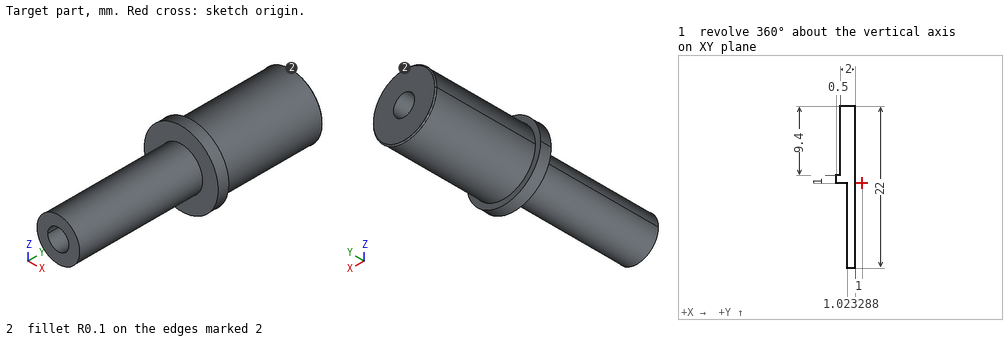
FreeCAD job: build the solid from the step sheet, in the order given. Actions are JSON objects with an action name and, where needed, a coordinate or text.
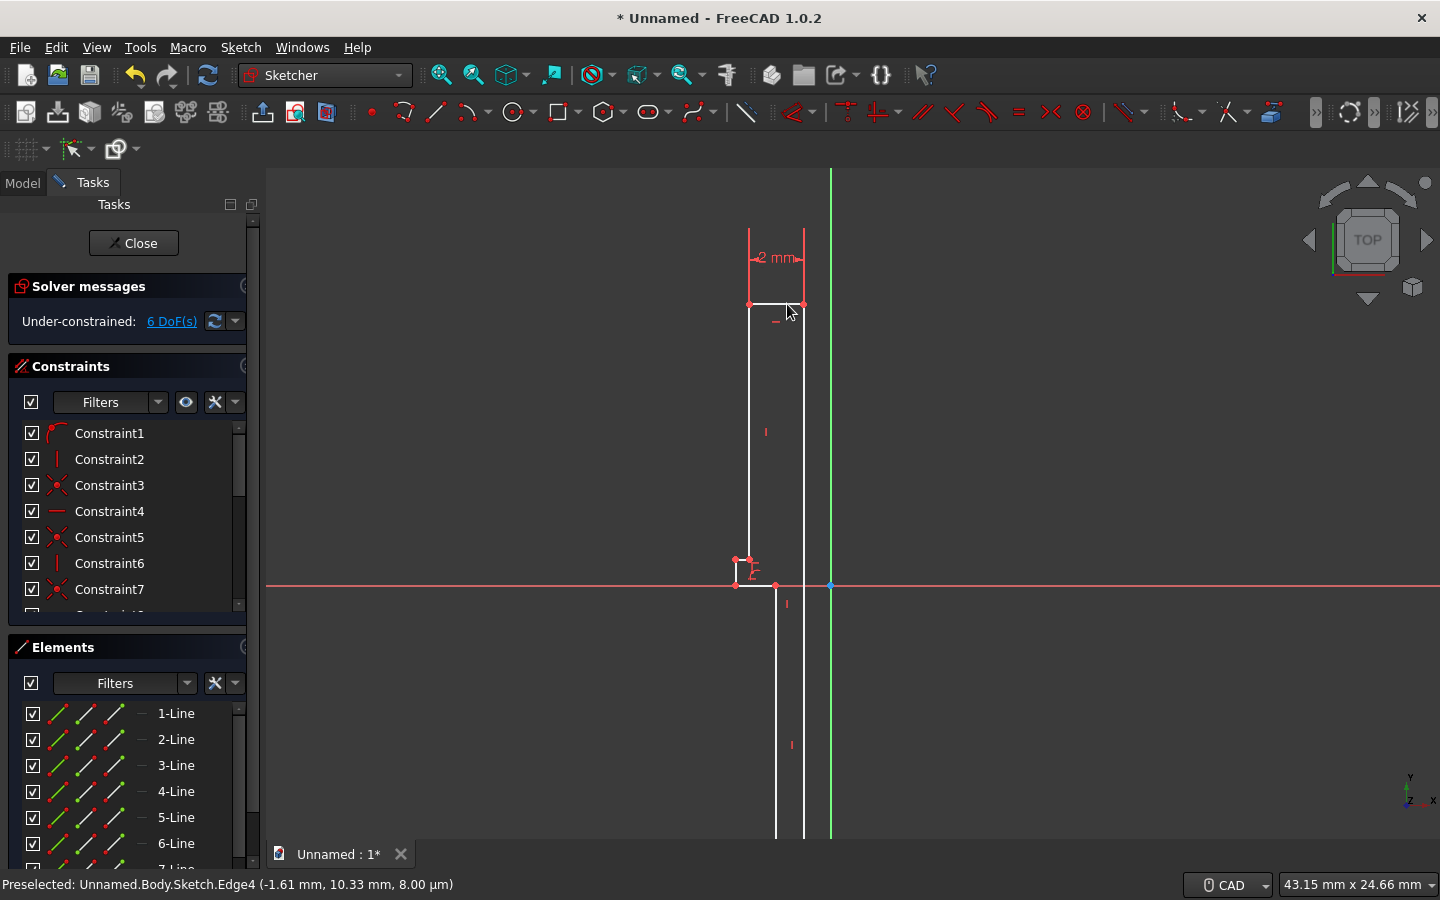
{"action": "scroll", "coordinate": [736, 570], "scroll_direction": "up", "scroll_amount": 2}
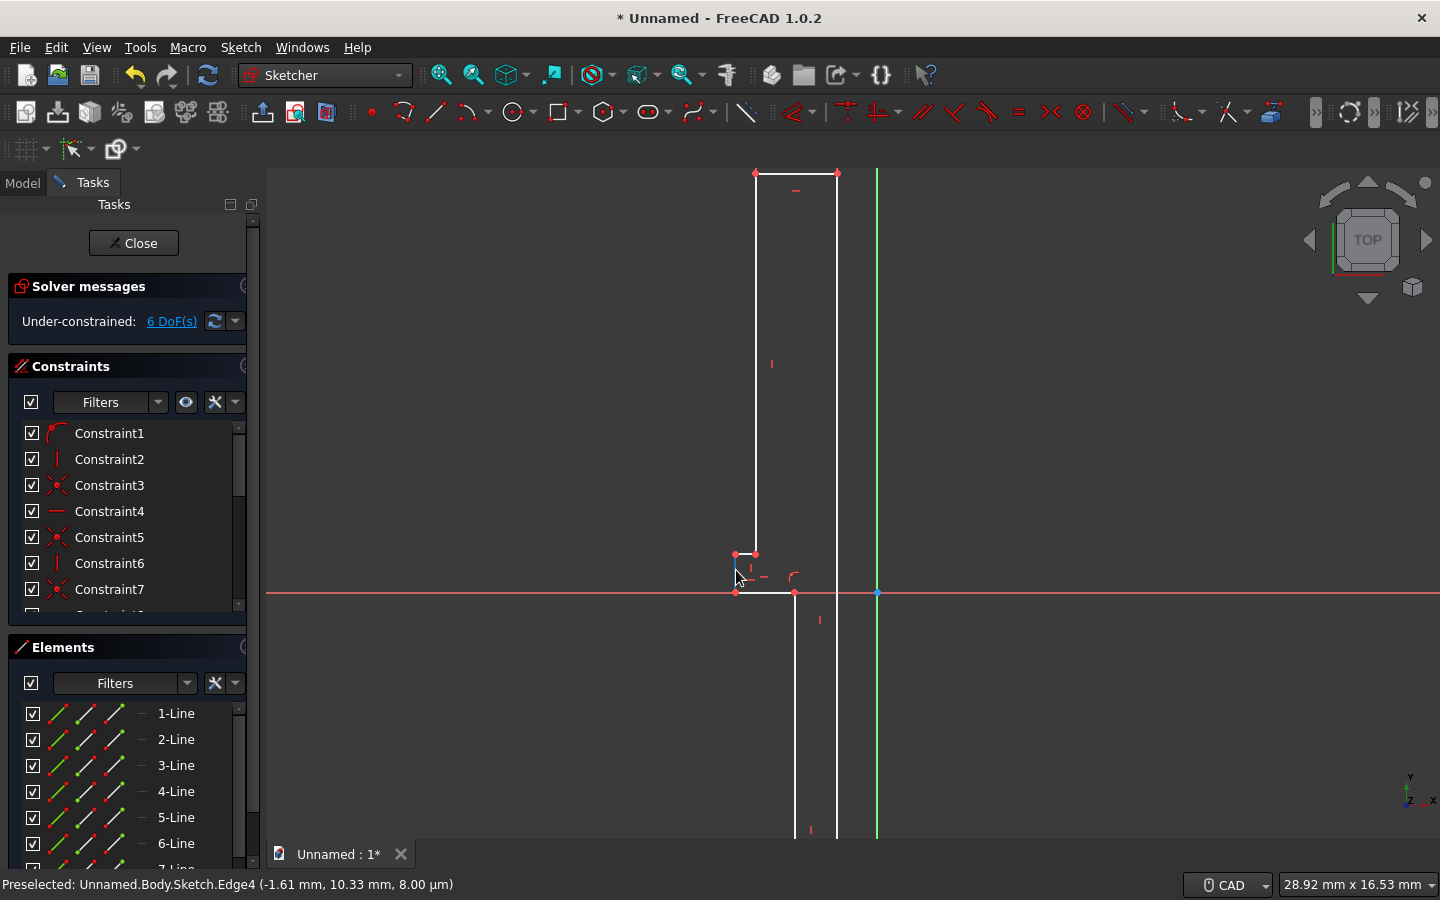
{"action": "left_click", "coordinate": [735, 570]}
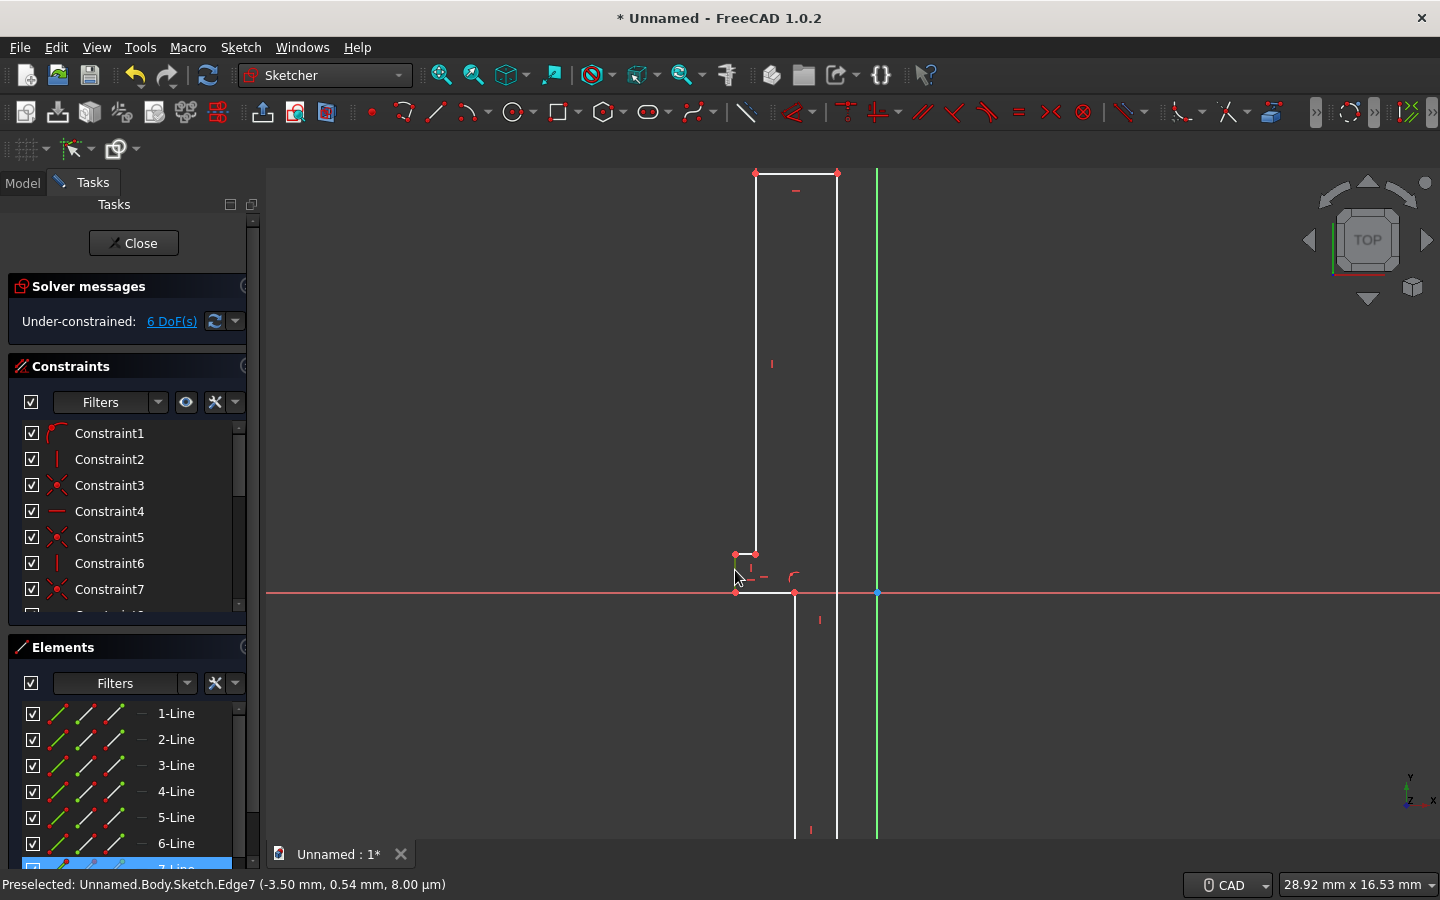
{"action": "key", "text": "i"}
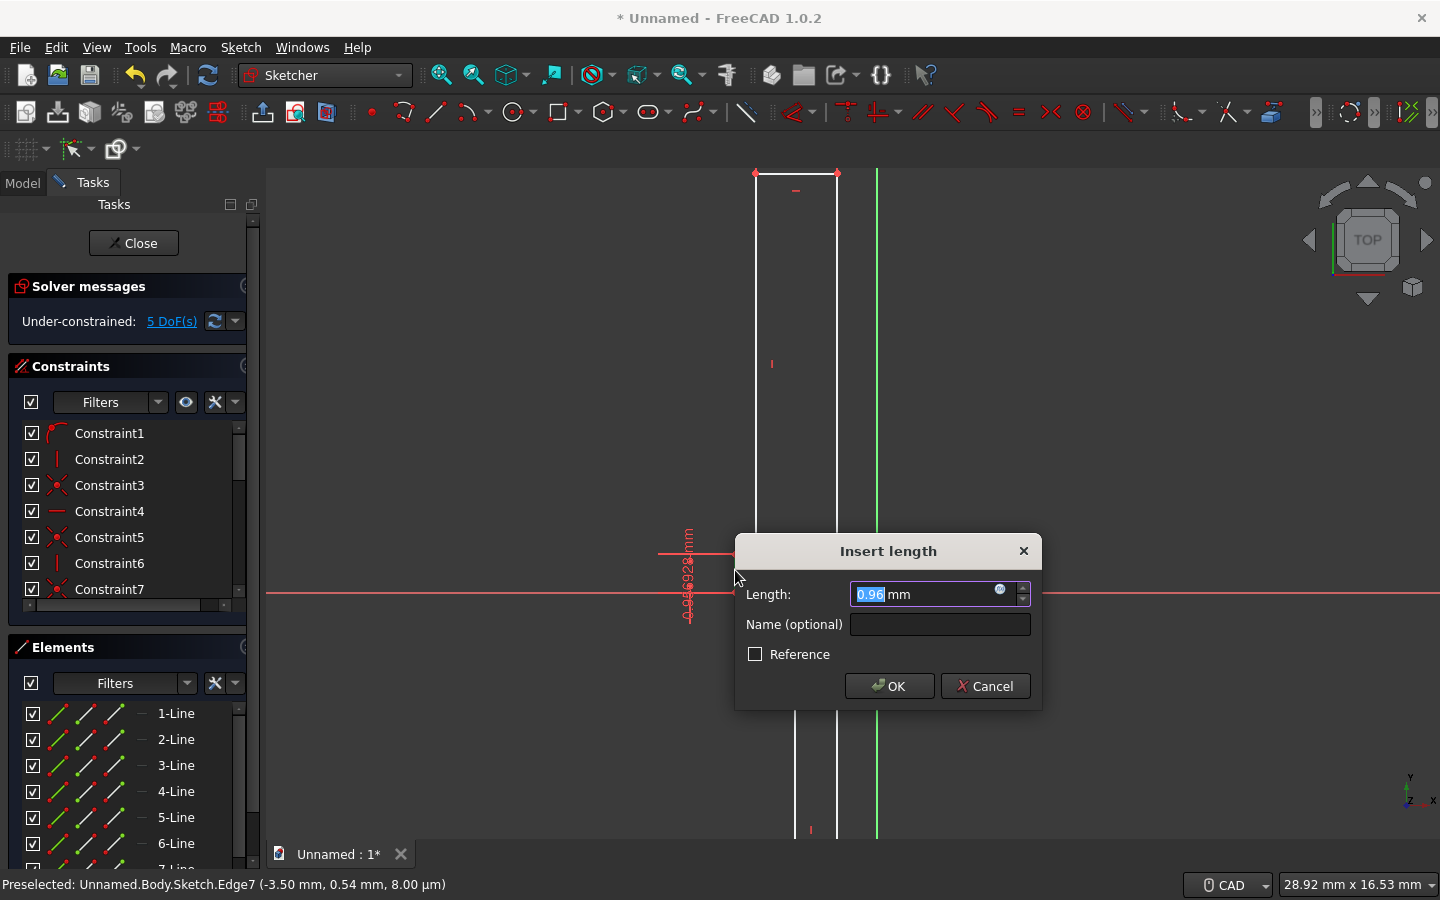
{"action": "type", "text": "1"}
{"action": "key", "text": "Return"}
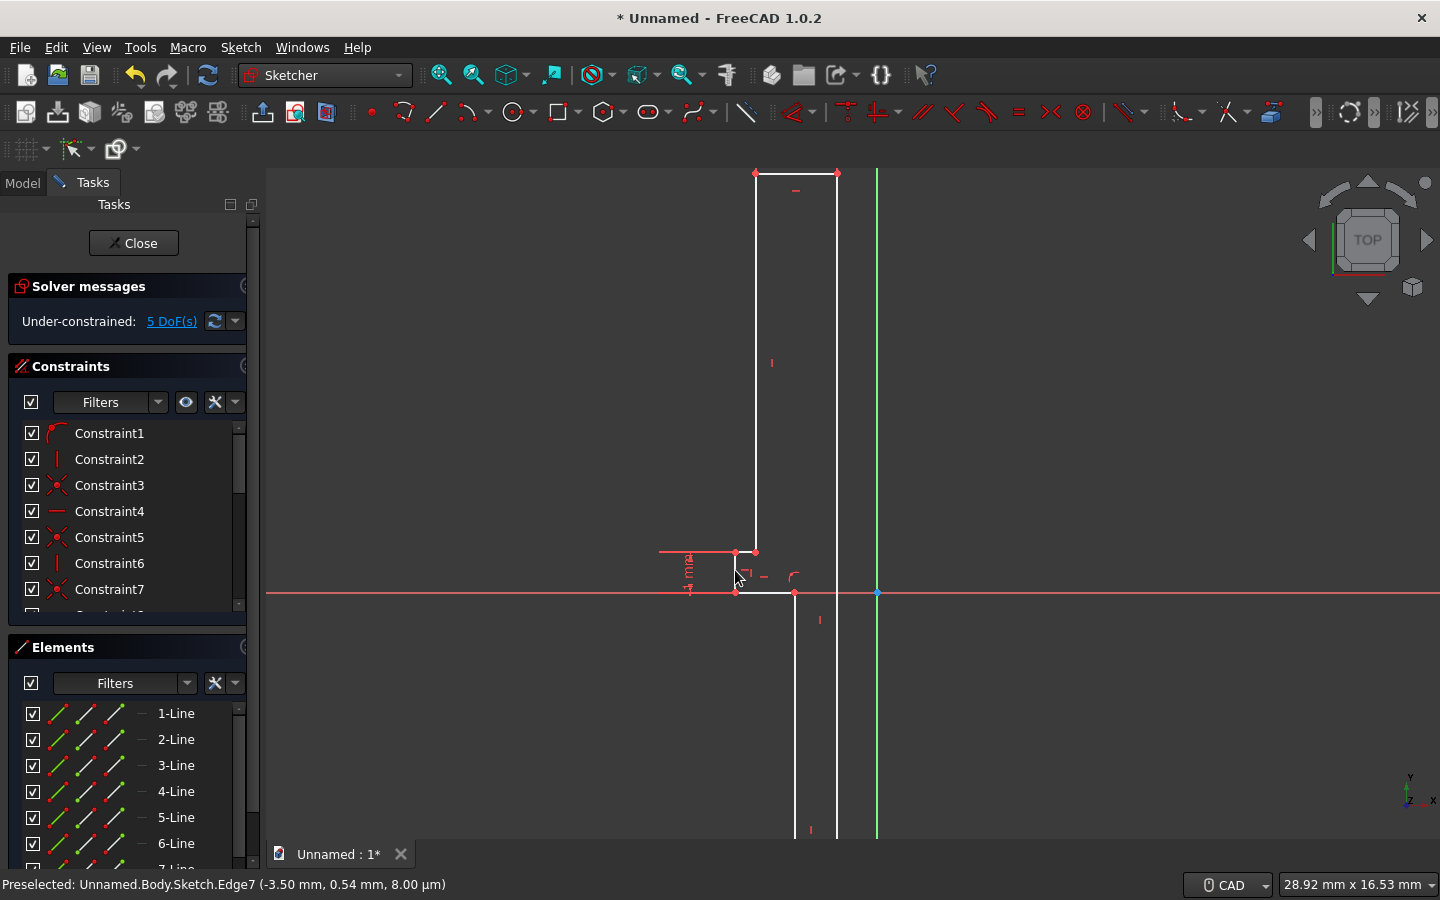
{"action": "left_click", "coordinate": [837, 798]}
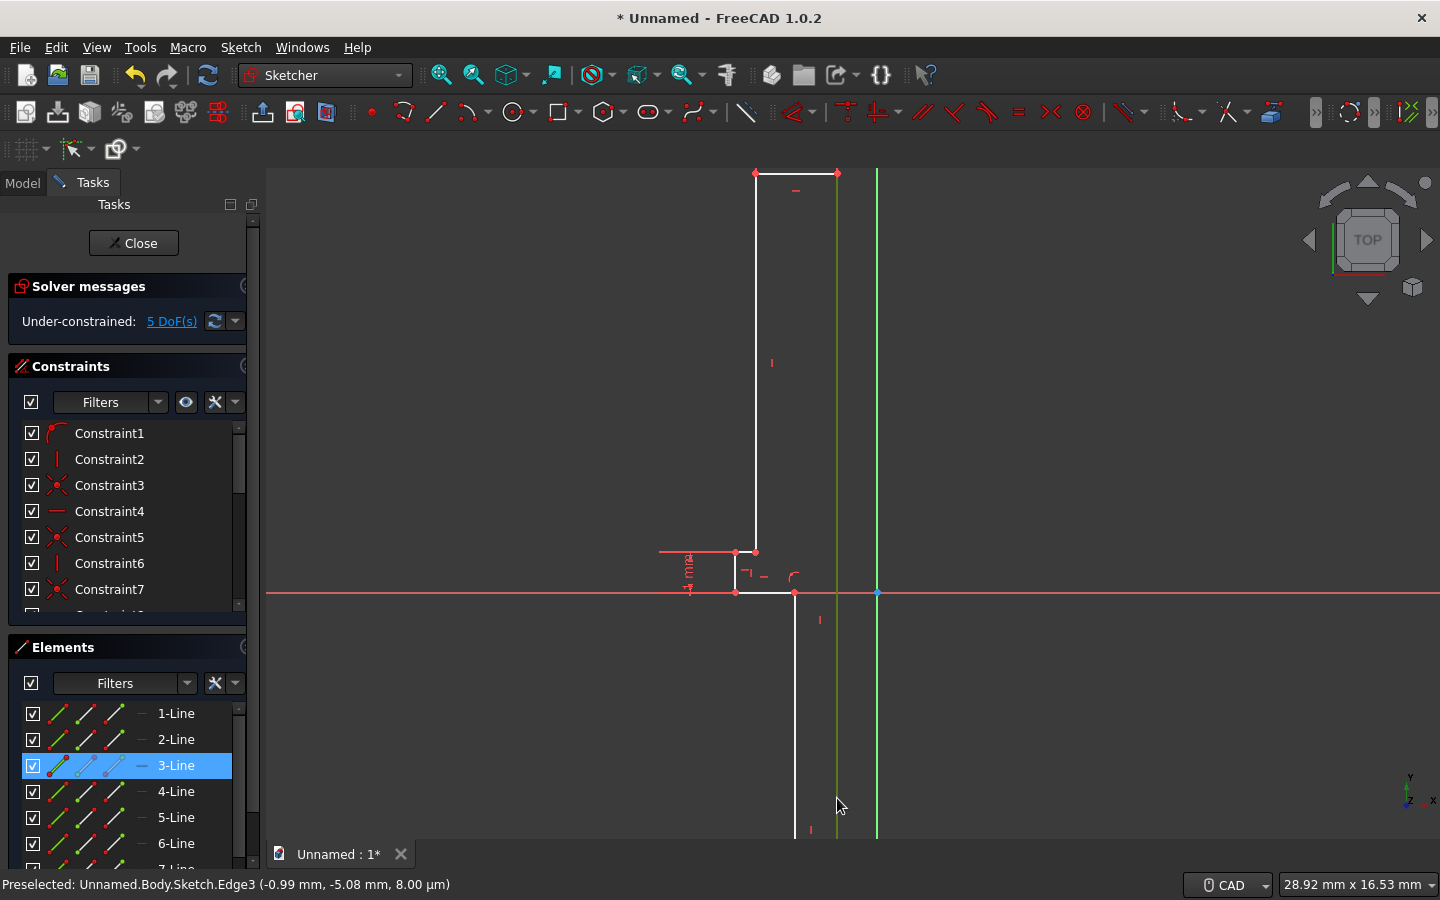
{"action": "left_click", "coordinate": [814, 112]}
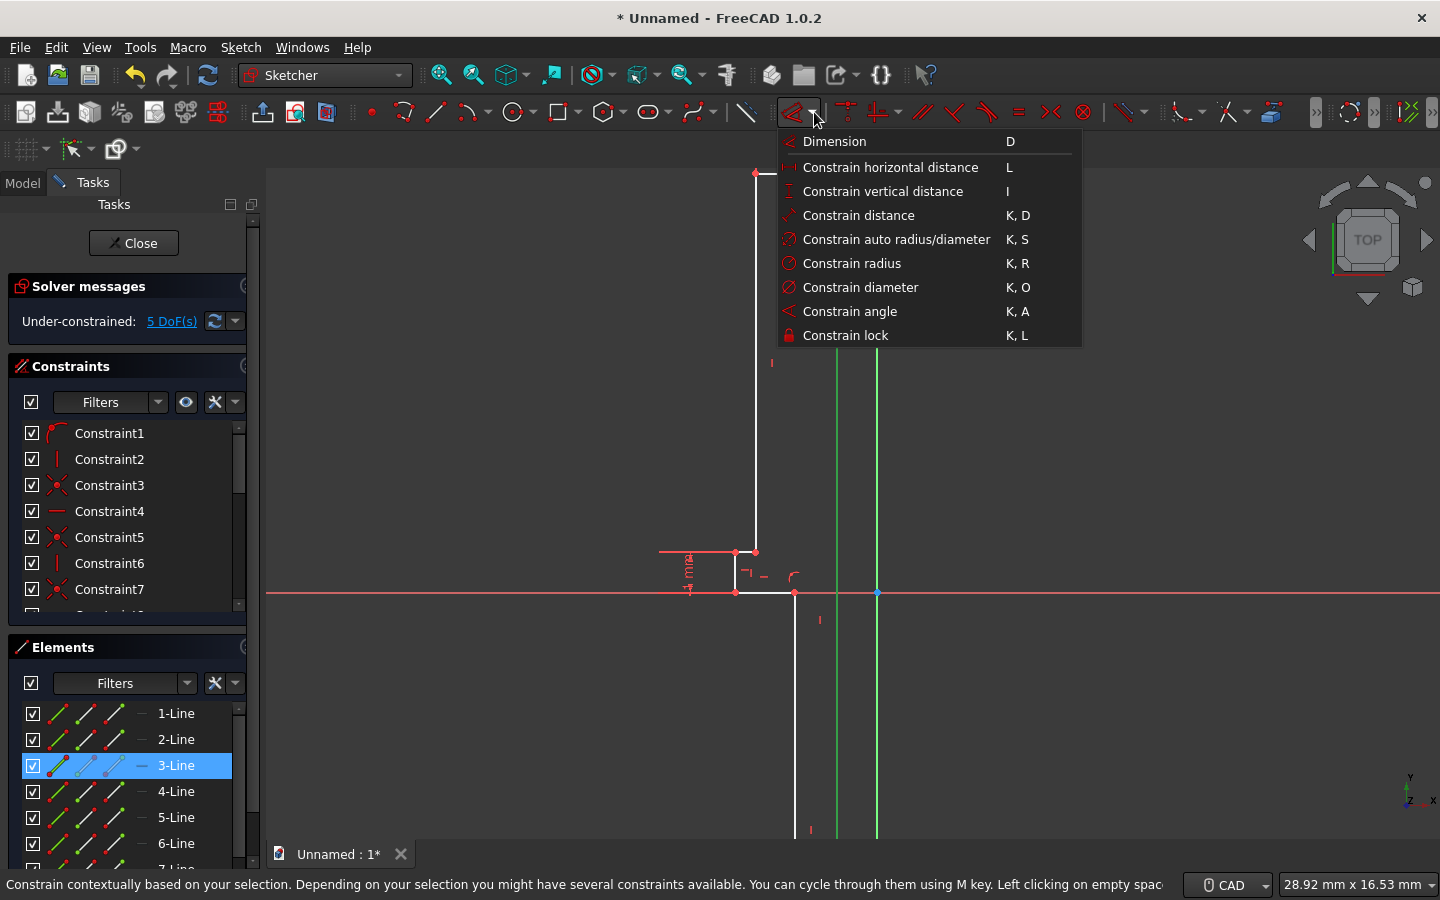
{"action": "left_click", "coordinate": [930, 191]}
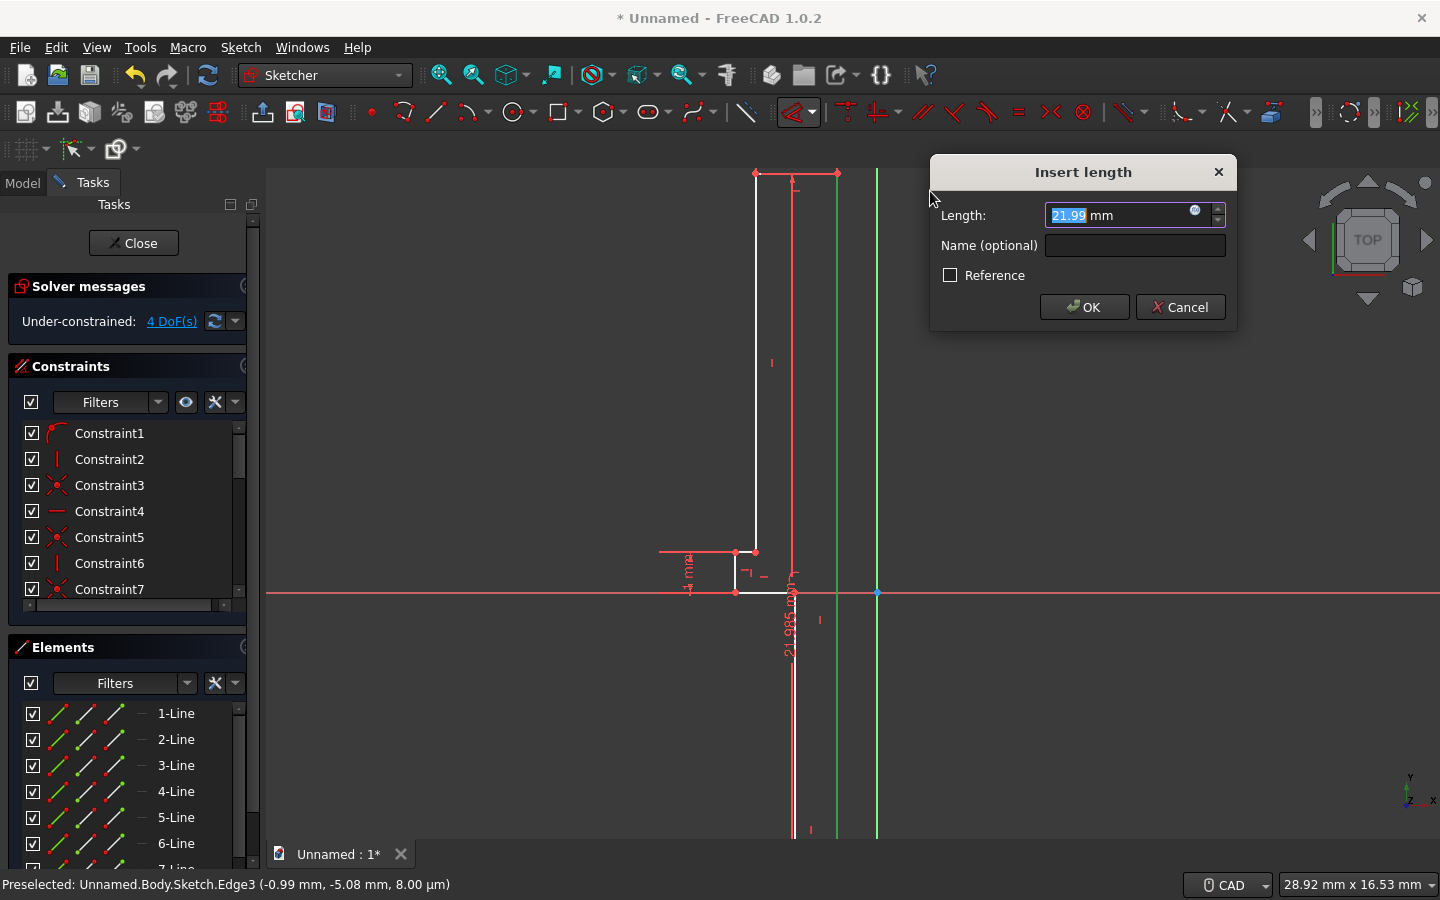
{"action": "type", "text": "22"}
{"action": "key", "text": "Return"}